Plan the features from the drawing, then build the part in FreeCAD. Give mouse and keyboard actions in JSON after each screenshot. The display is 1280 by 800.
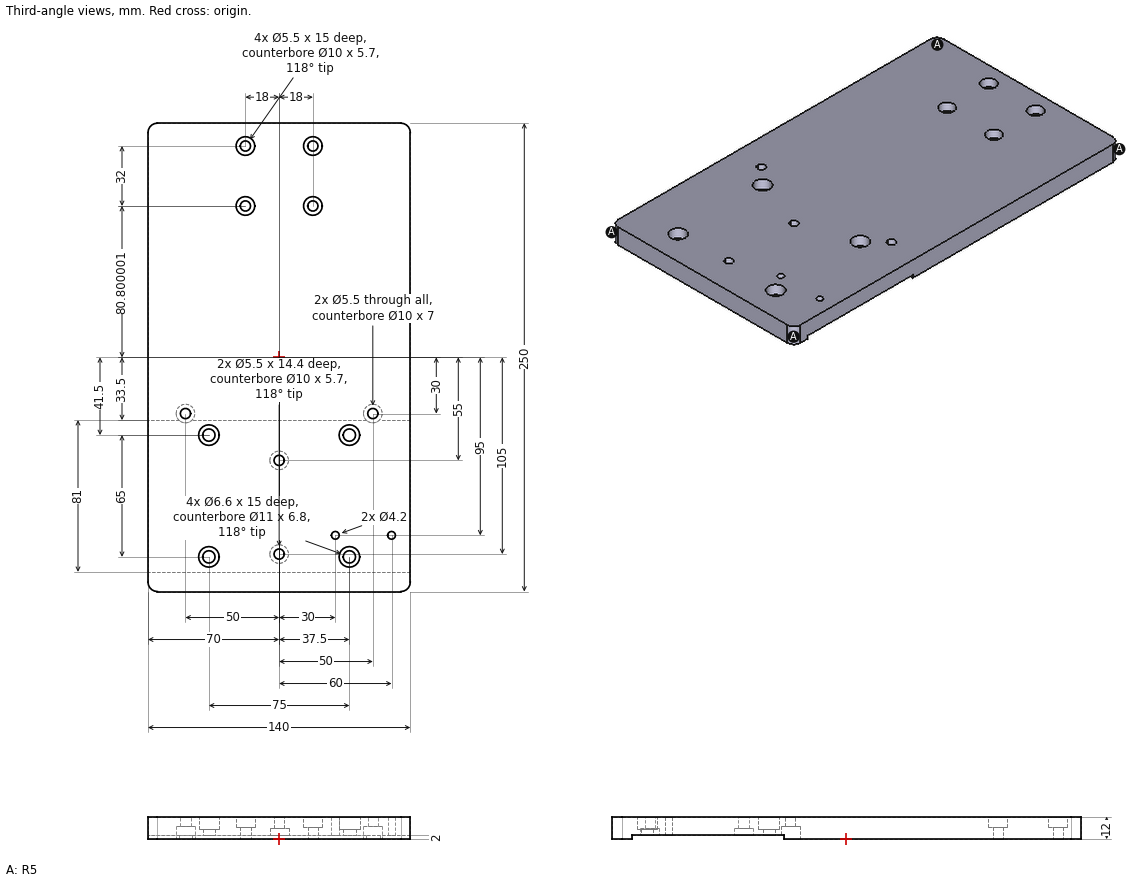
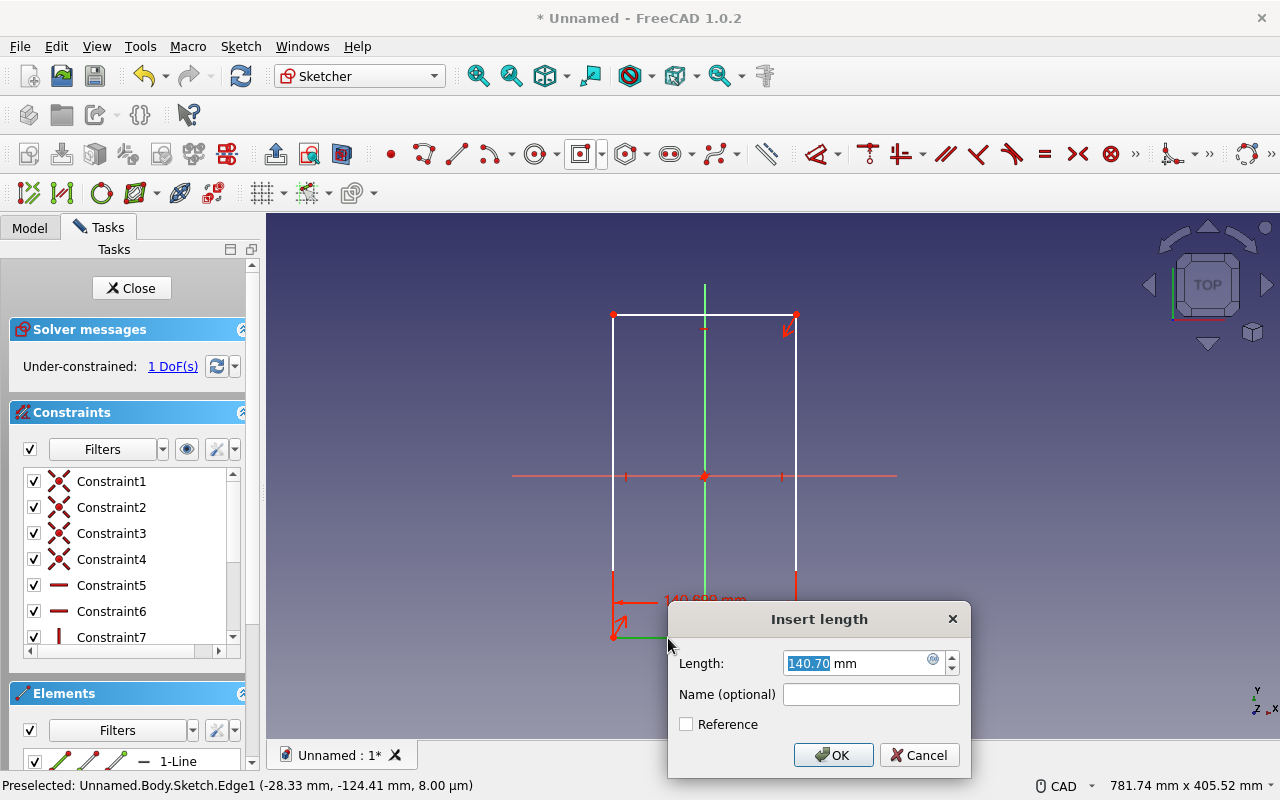
{"action": "type", "text": "140"}
{"action": "key", "text": "Return"}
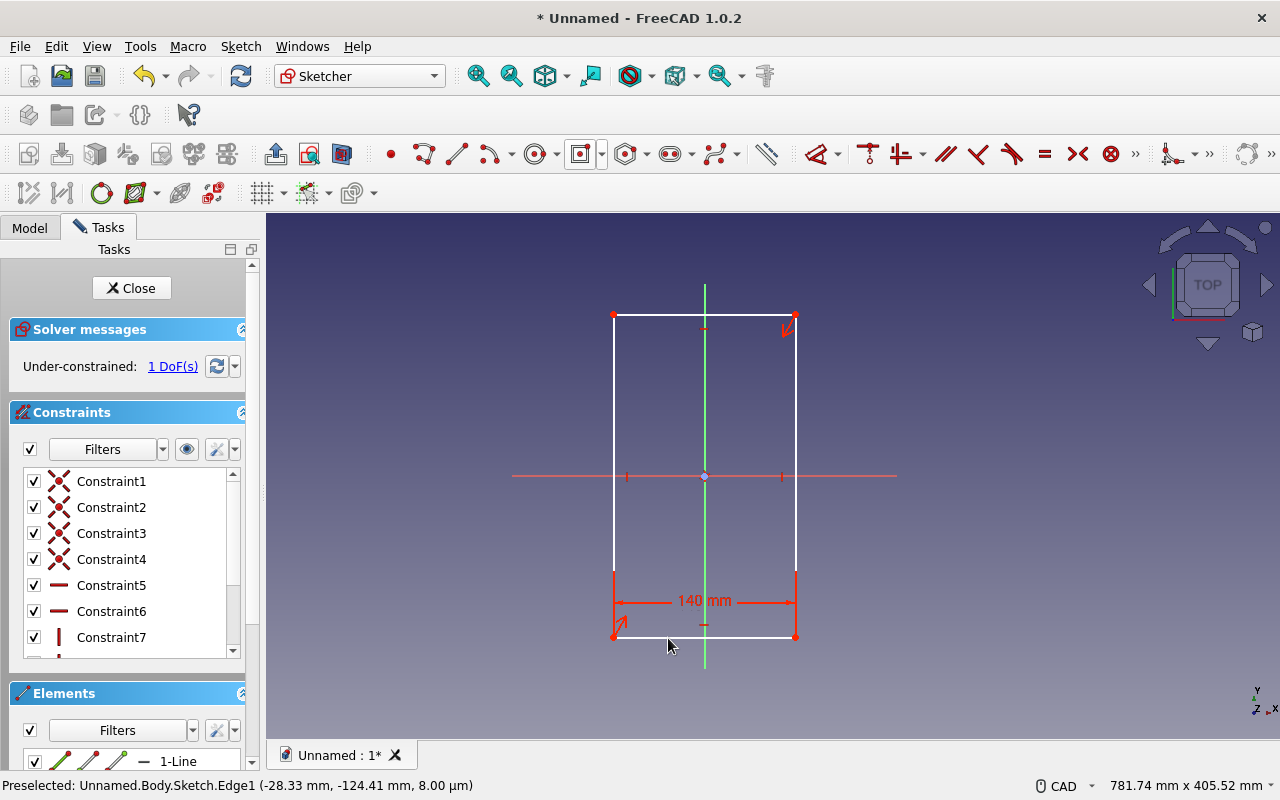
{"action": "left_click", "coordinate": [796, 541]}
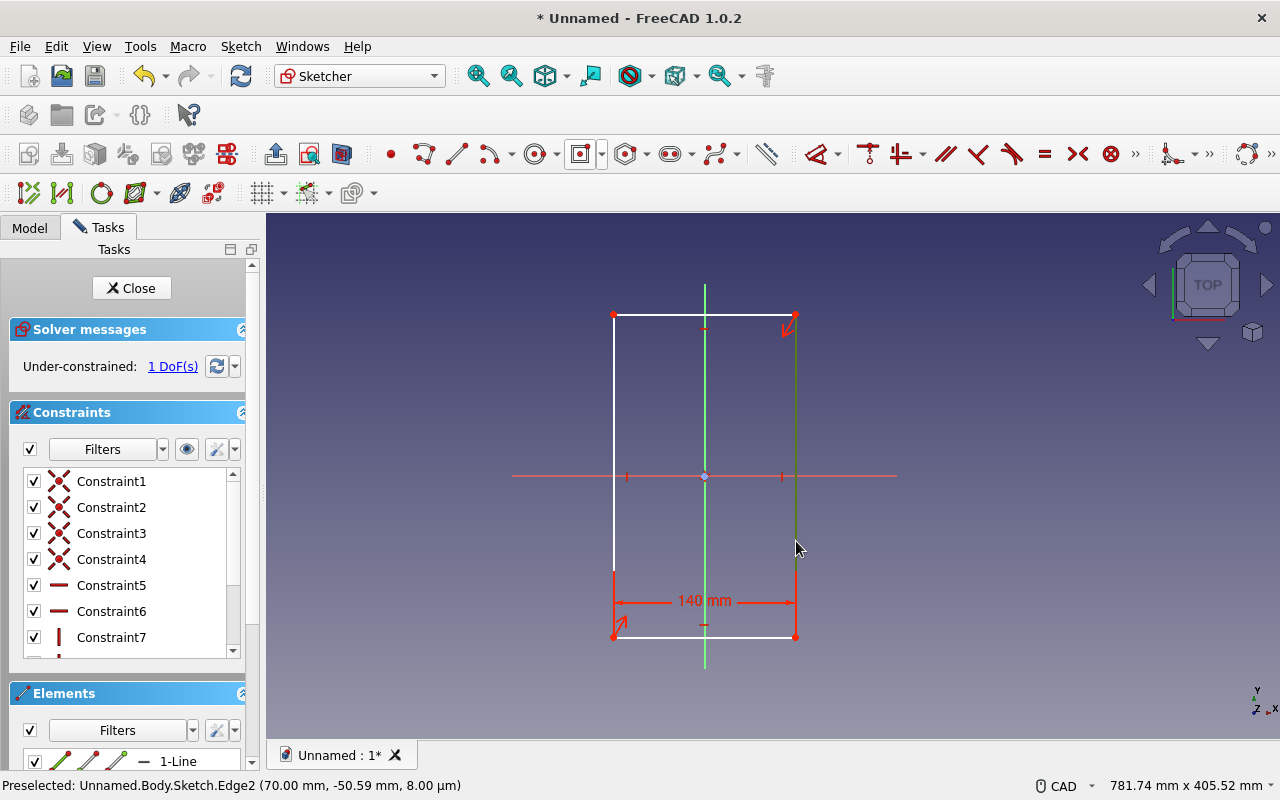
{"action": "key", "text": "i"}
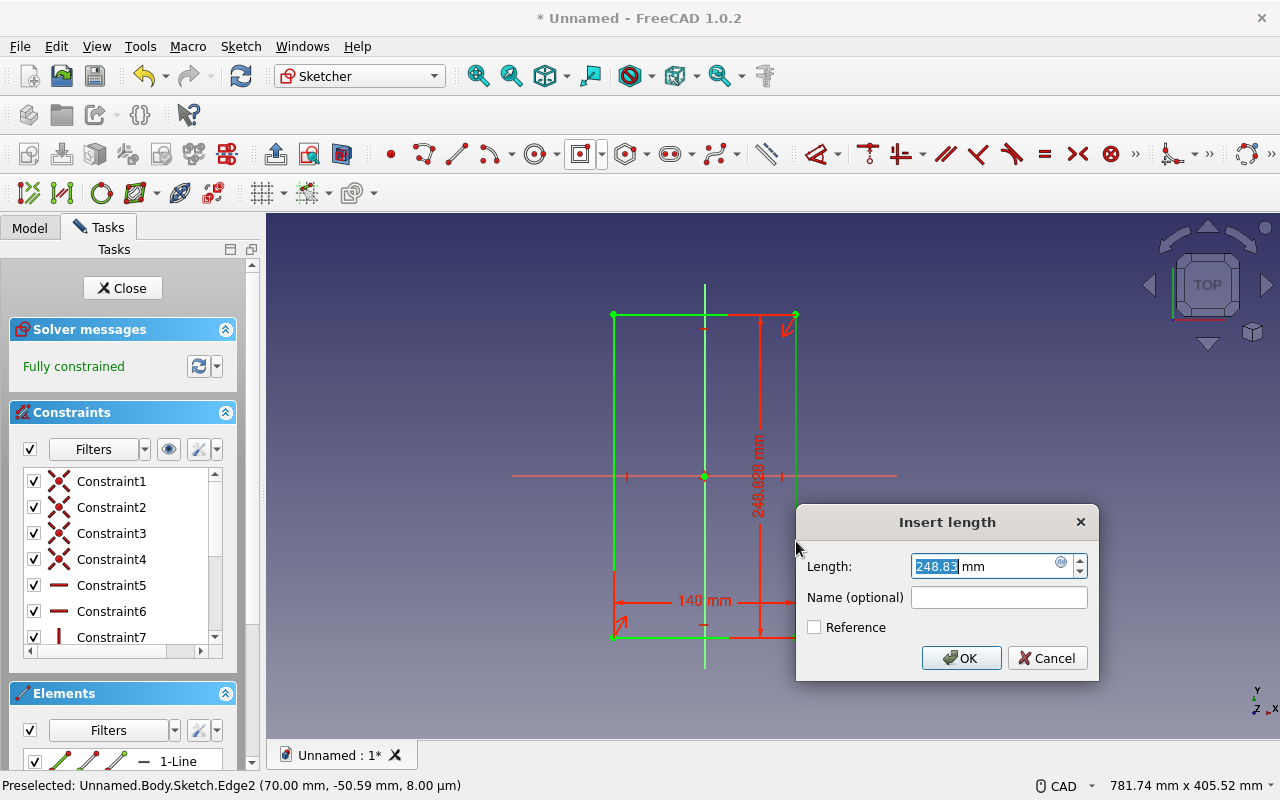
{"action": "type", "text": "250"}
{"action": "key", "text": "Return"}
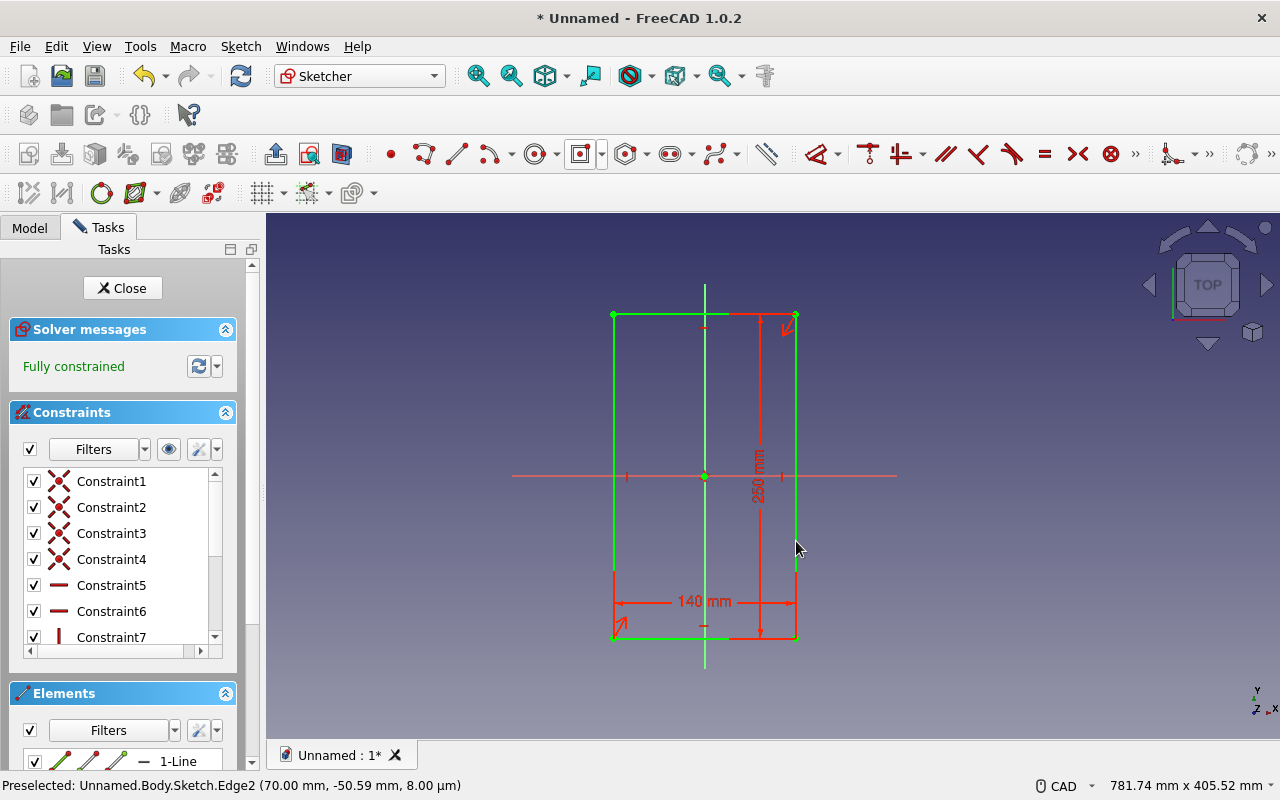
{"action": "left_click", "coordinate": [123, 288]}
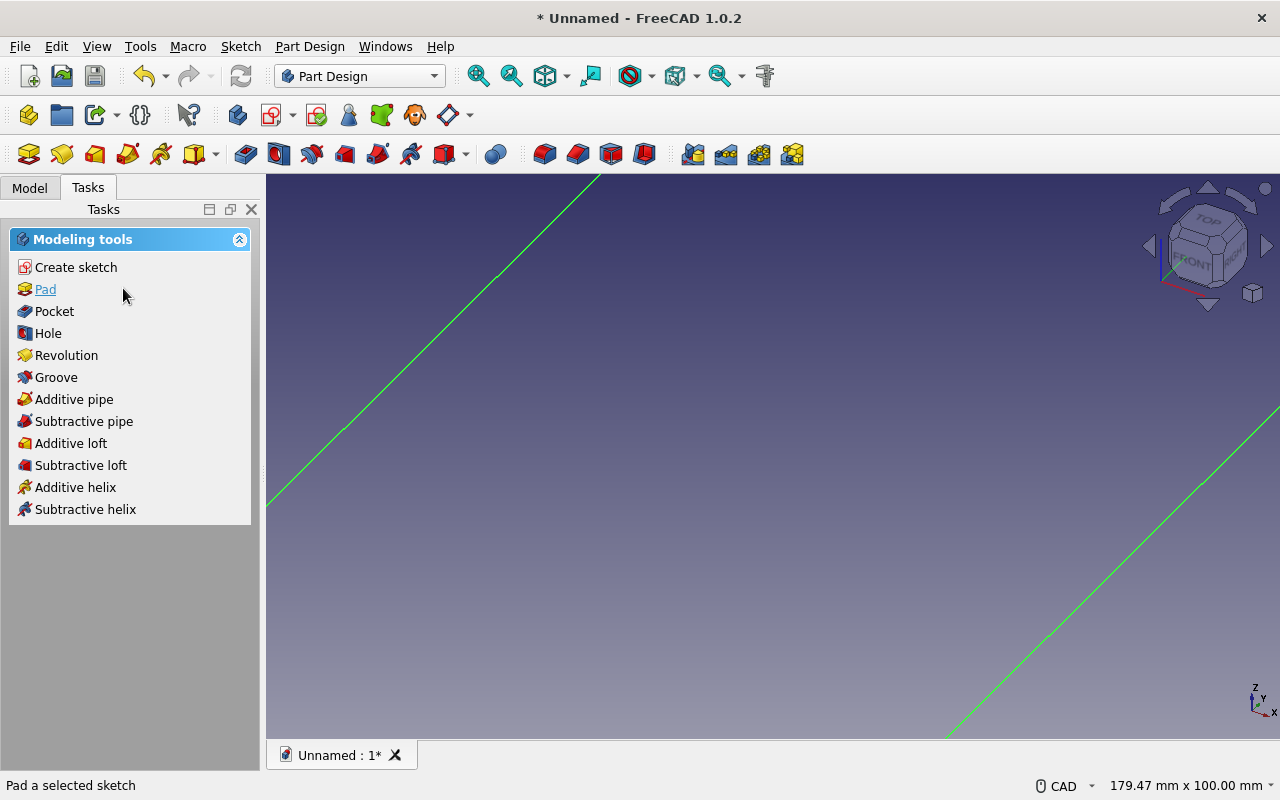
{"action": "left_click", "coordinate": [29, 154]}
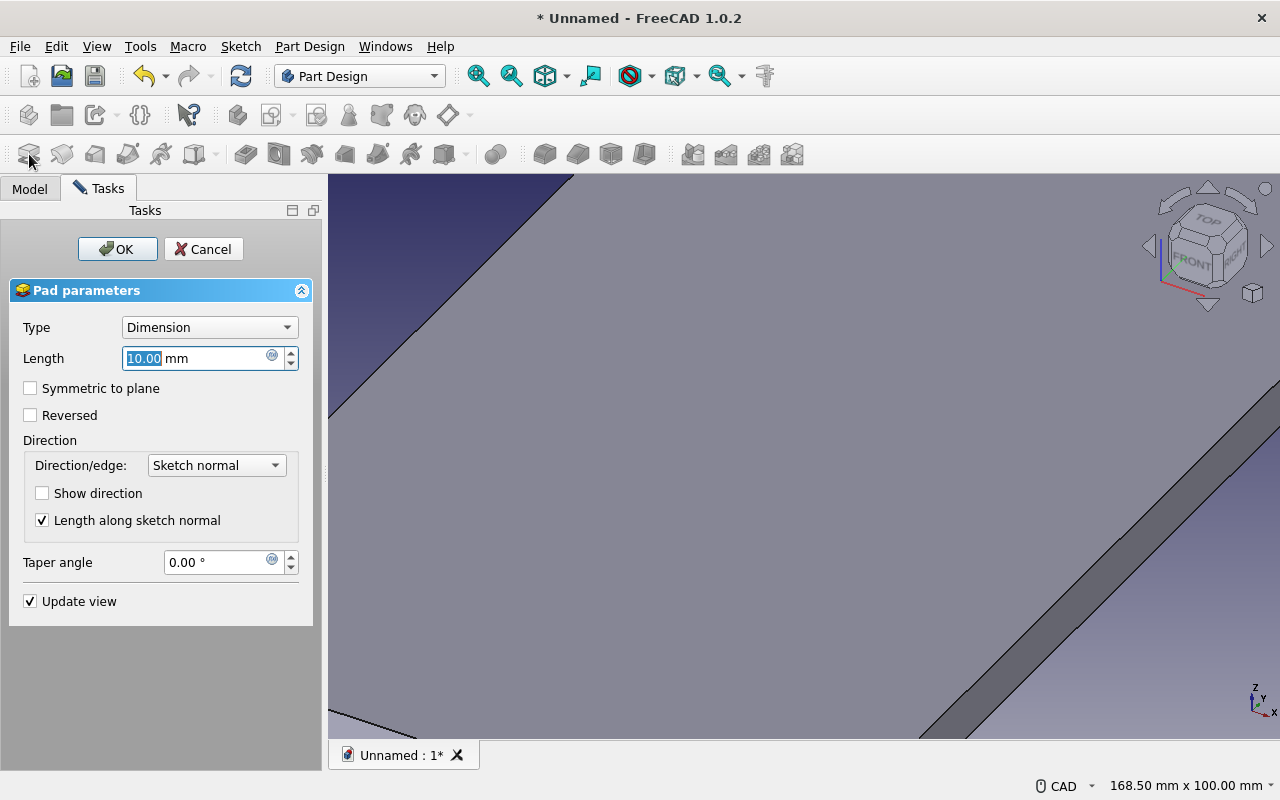
{"action": "type", "text": "12"}
{"action": "key", "text": "Tab"}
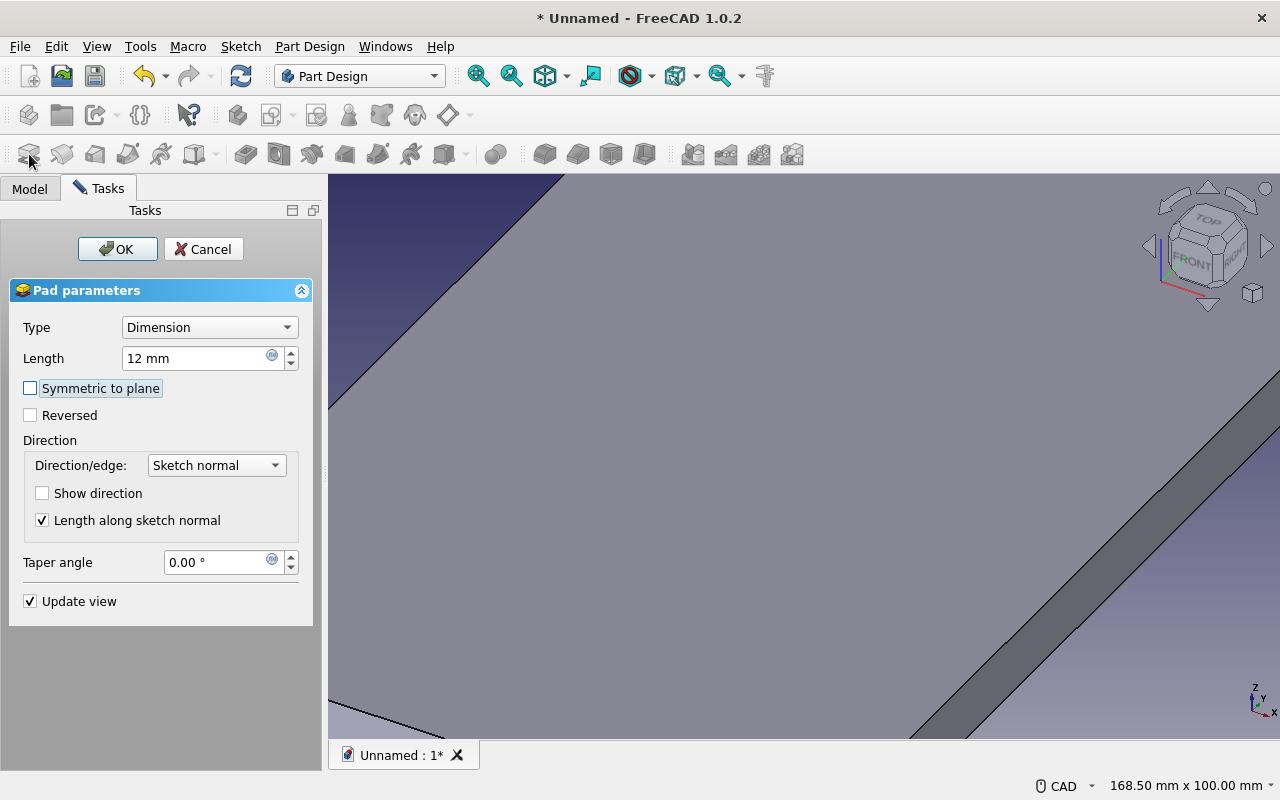
{"action": "left_click", "coordinate": [118, 249]}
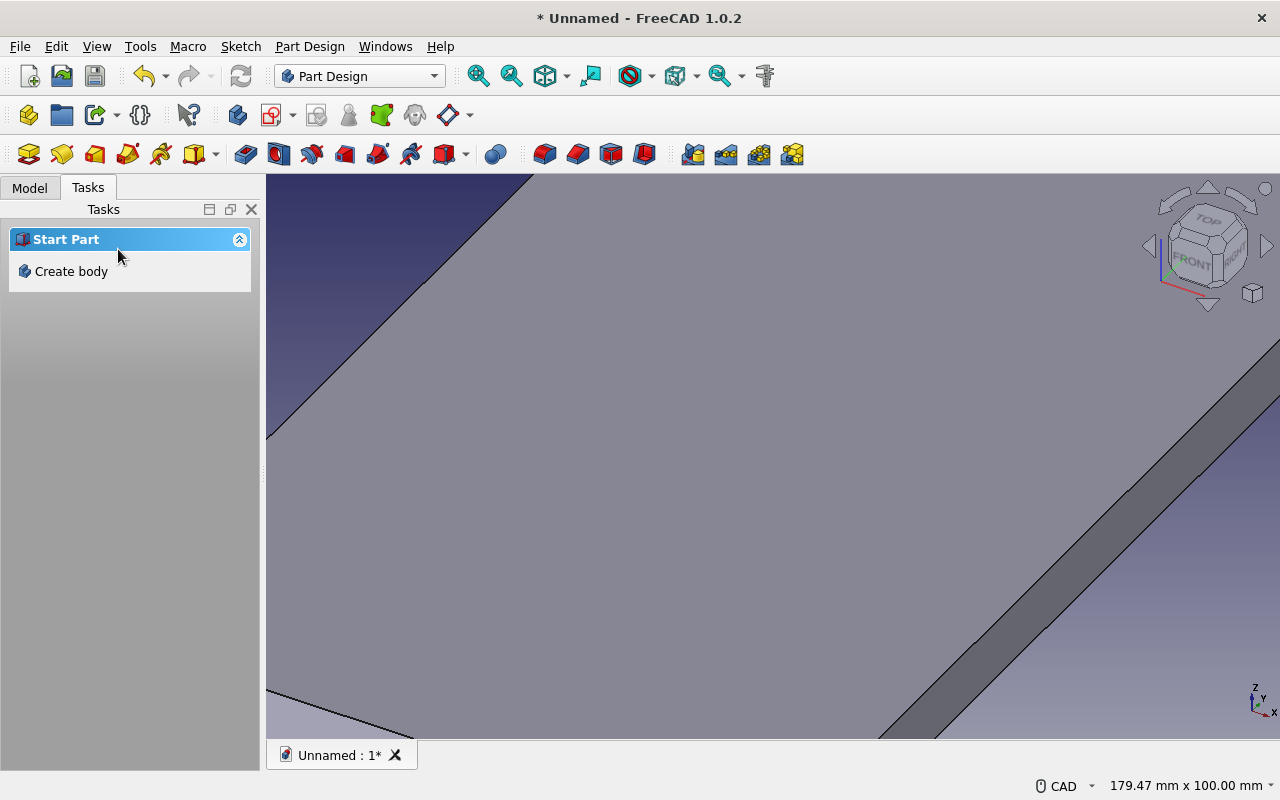
{"action": "left_click", "coordinate": [479, 76]}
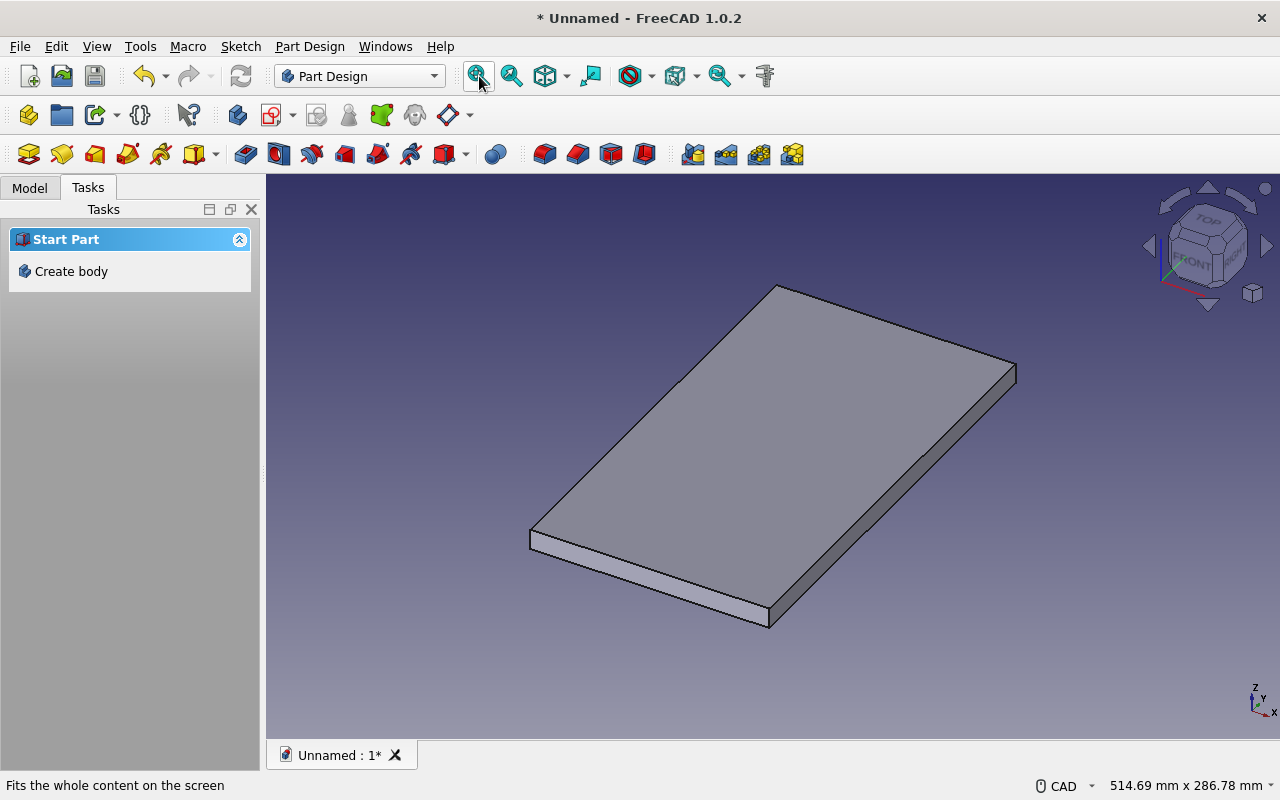
{"action": "left_click", "coordinate": [808, 411]}